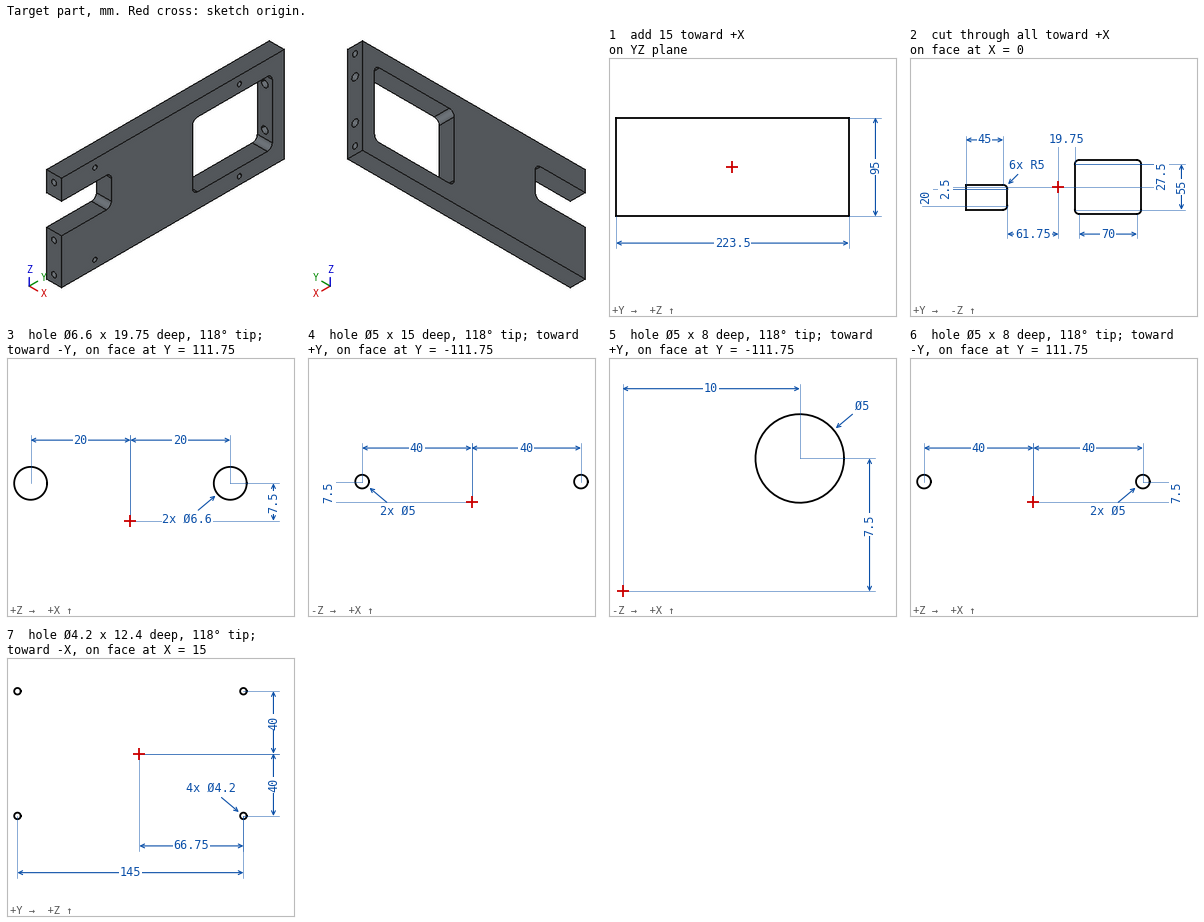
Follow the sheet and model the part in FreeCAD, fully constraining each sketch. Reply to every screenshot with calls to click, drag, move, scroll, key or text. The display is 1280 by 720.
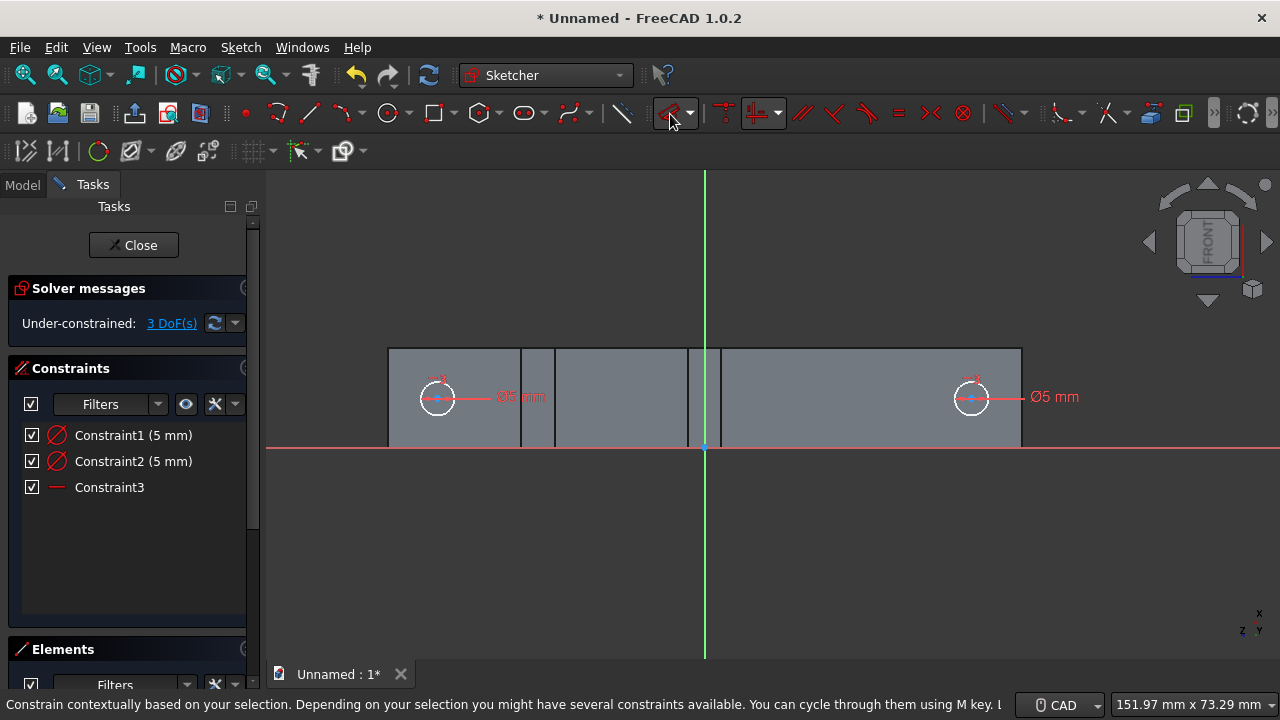
click(438, 399)
click(571, 482)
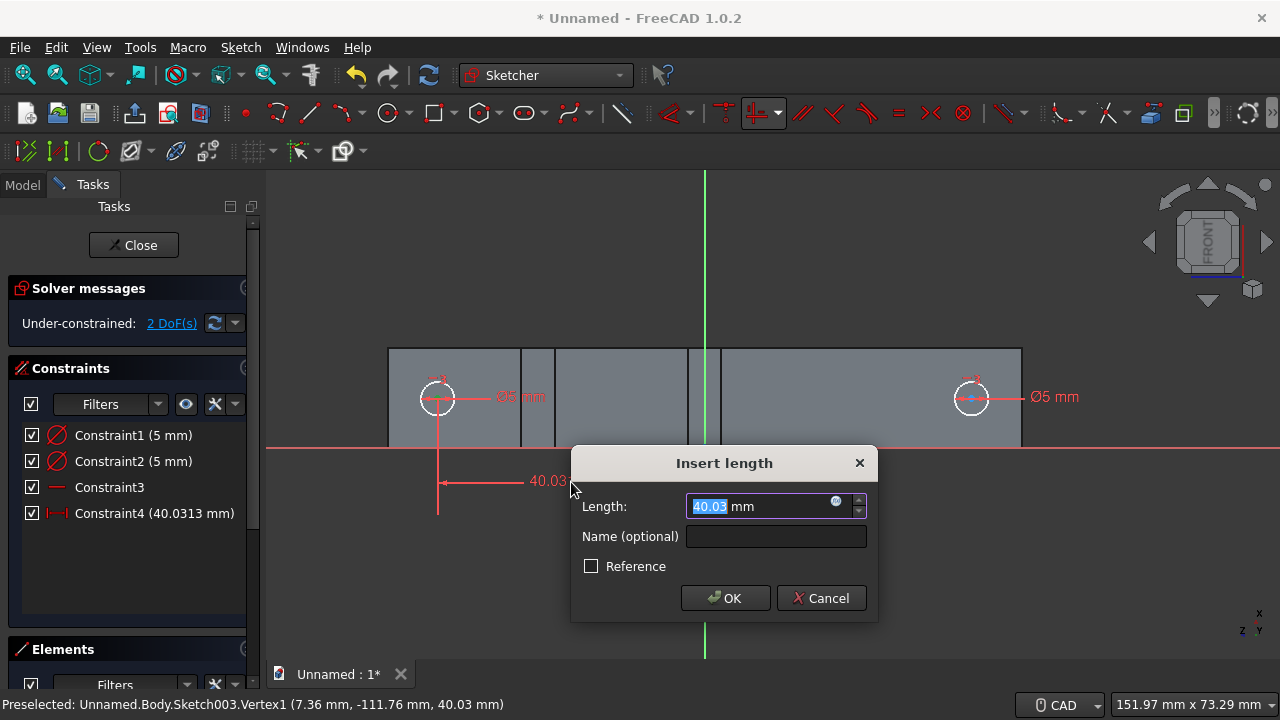
text(40)
key(Return)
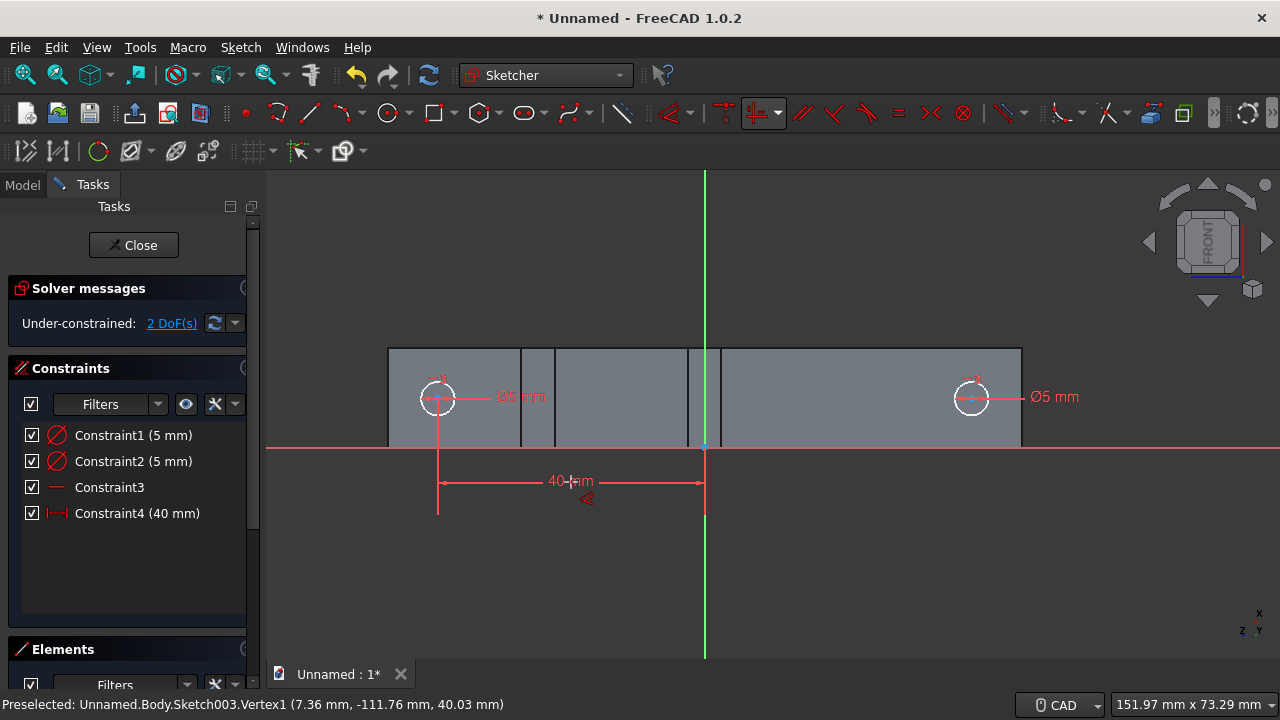
click(972, 399)
click(838, 482)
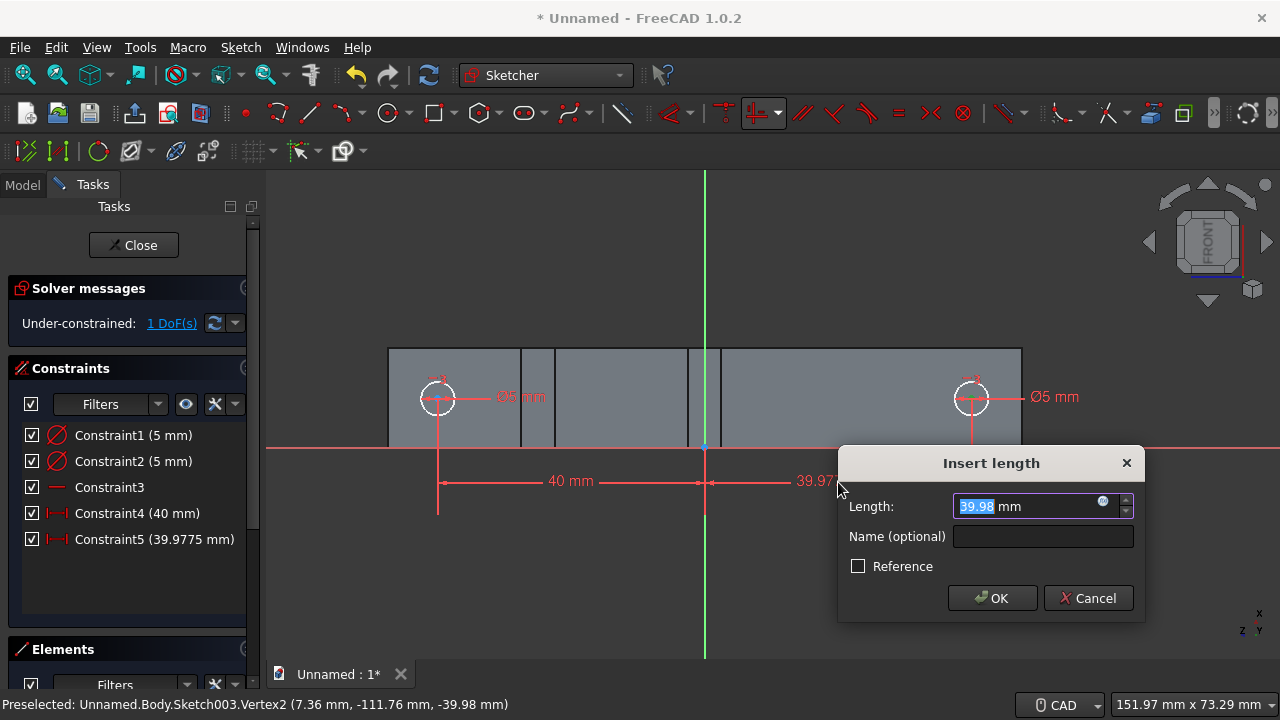
text(40)
key(Return)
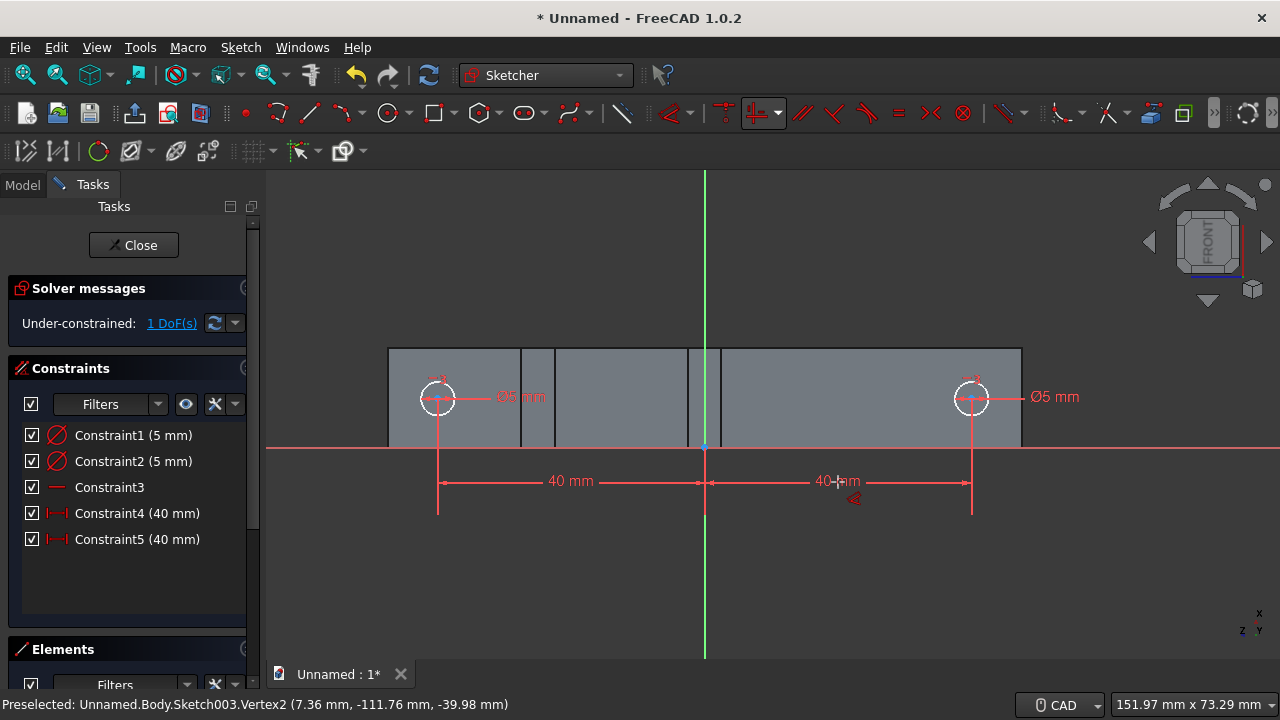
click(438, 399)
click(404, 423)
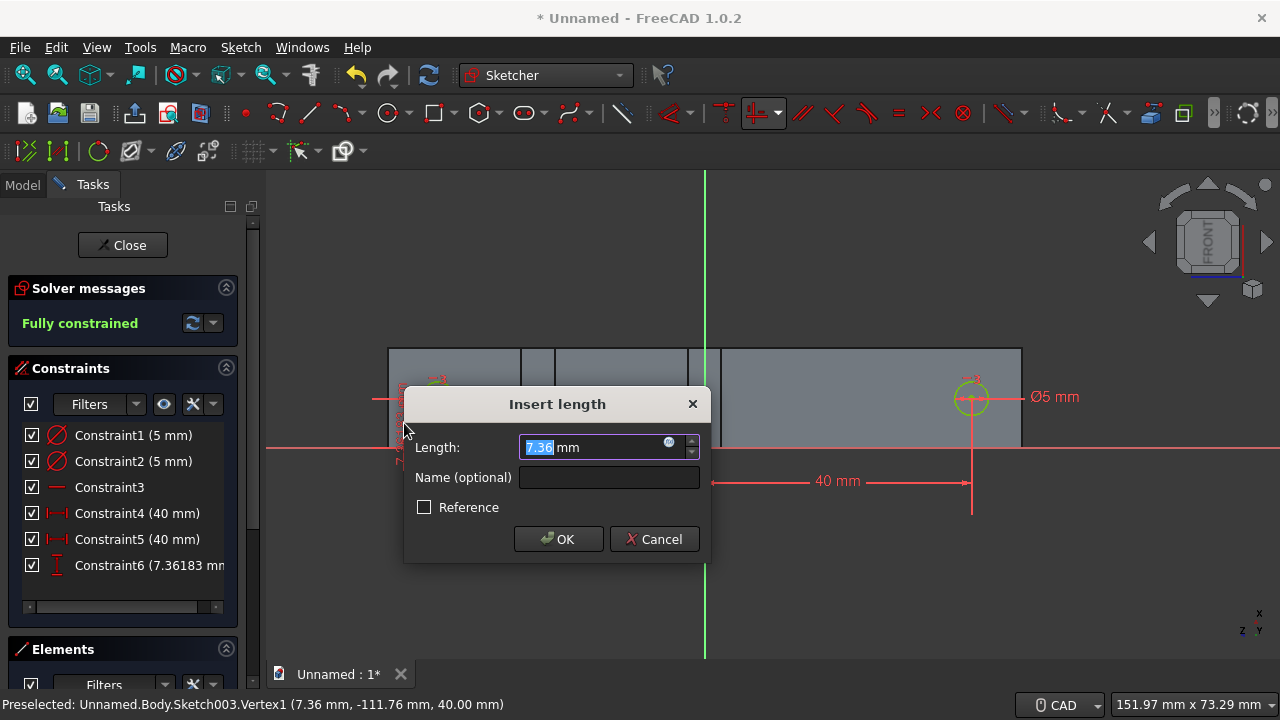
text(7.5)
key(Return)
key(Escape)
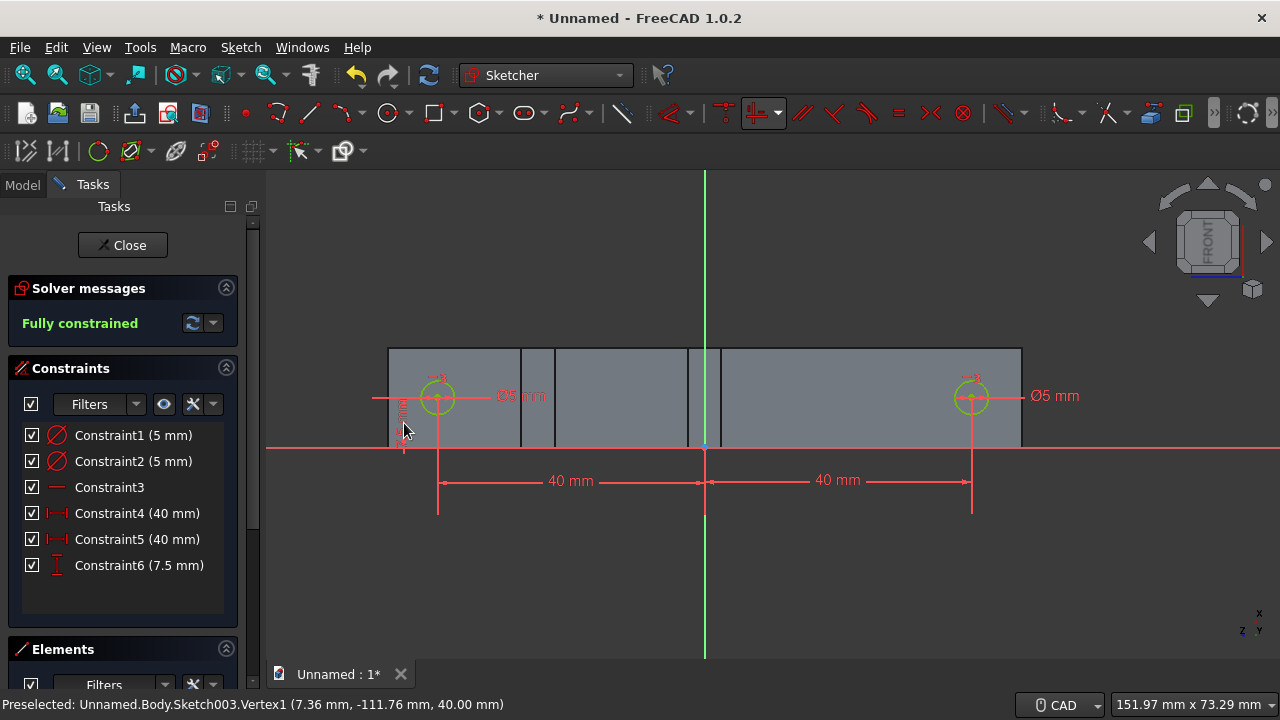
click(123, 245)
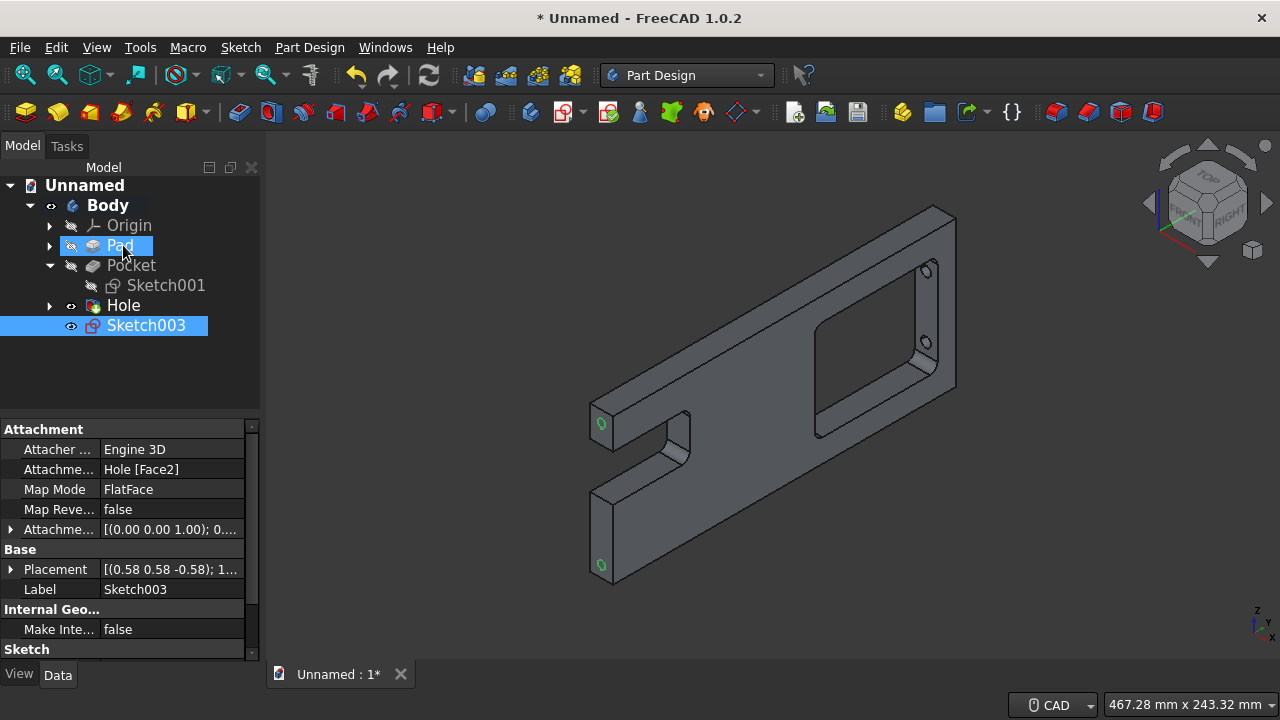
click(272, 112)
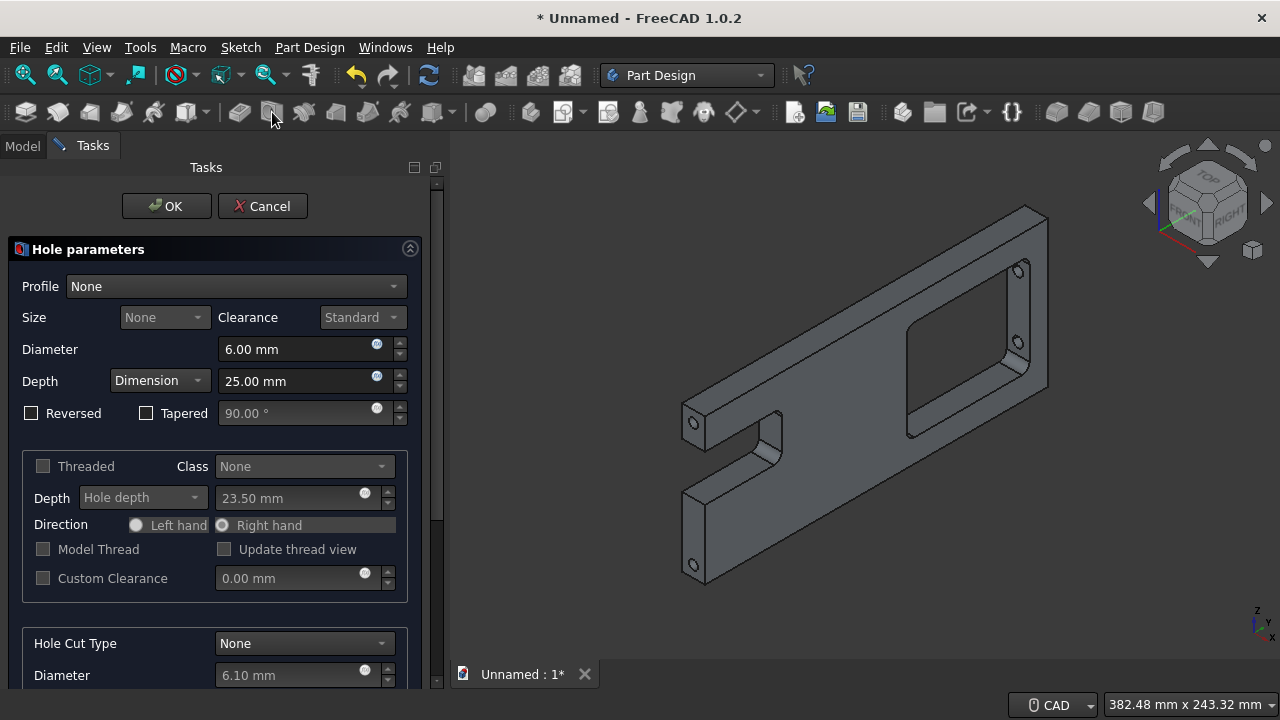
triple_click(305, 349)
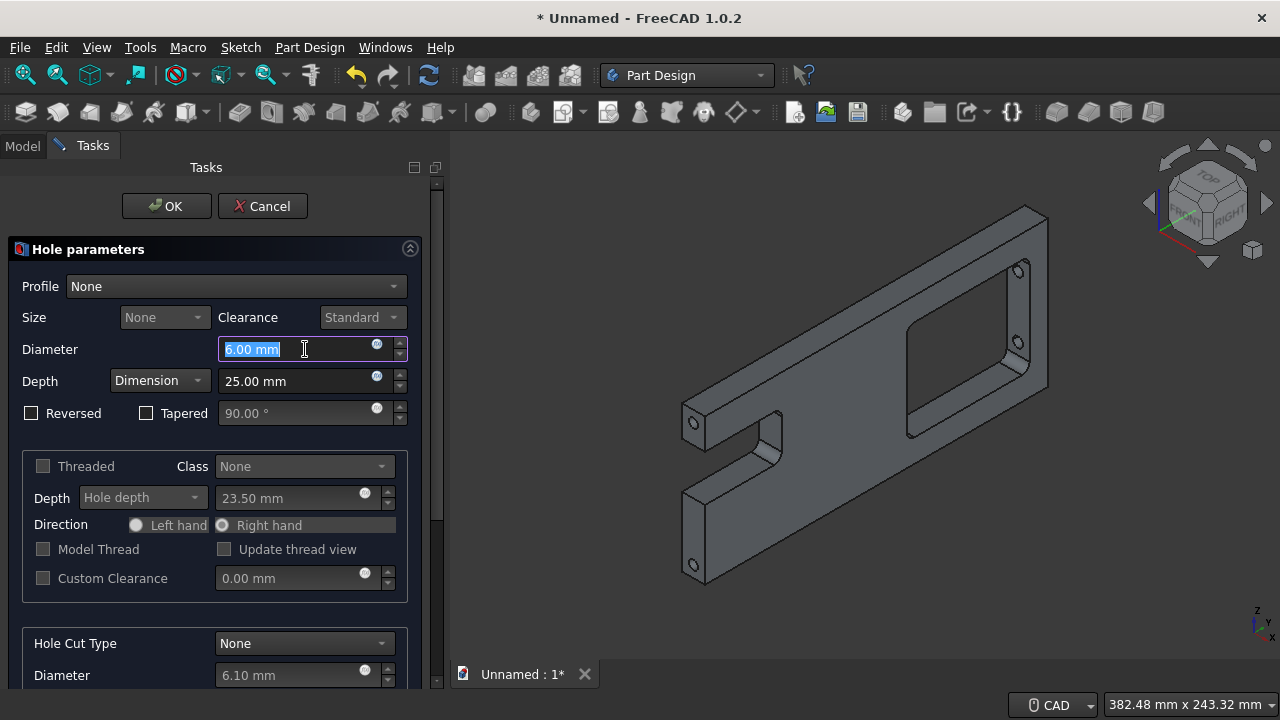
text(5)
key(Tab)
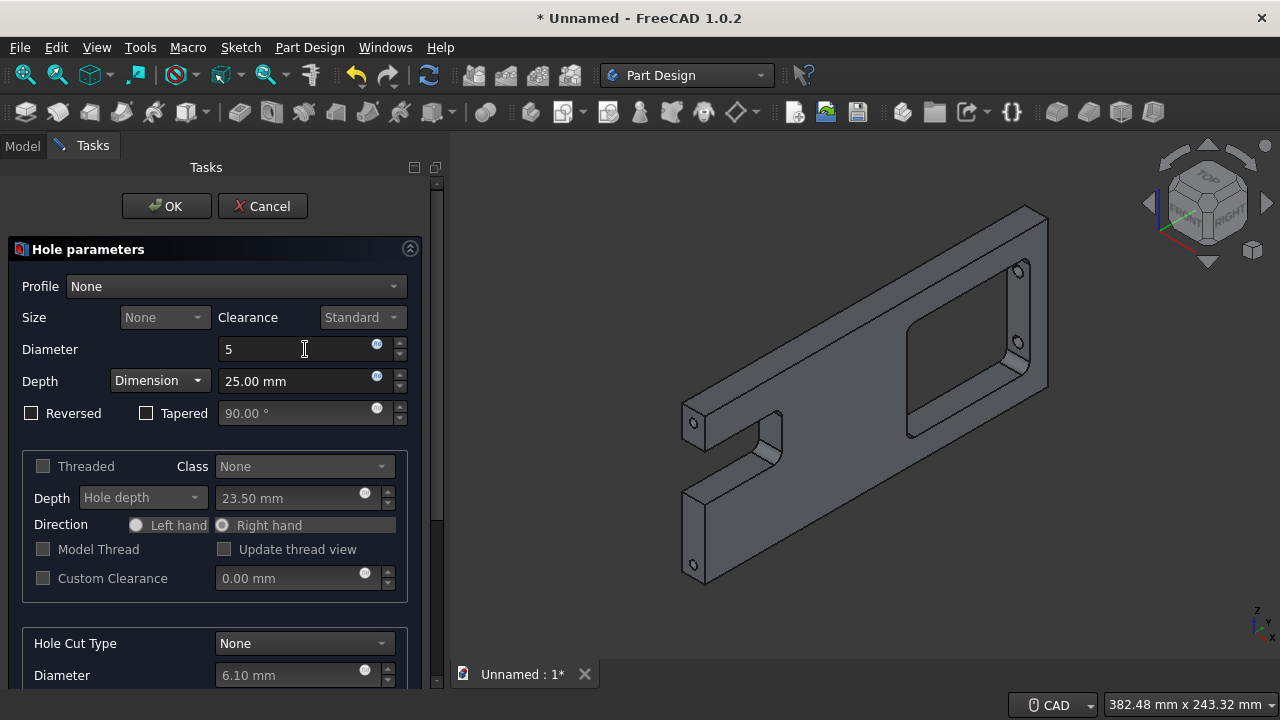
triple_click(305, 381)